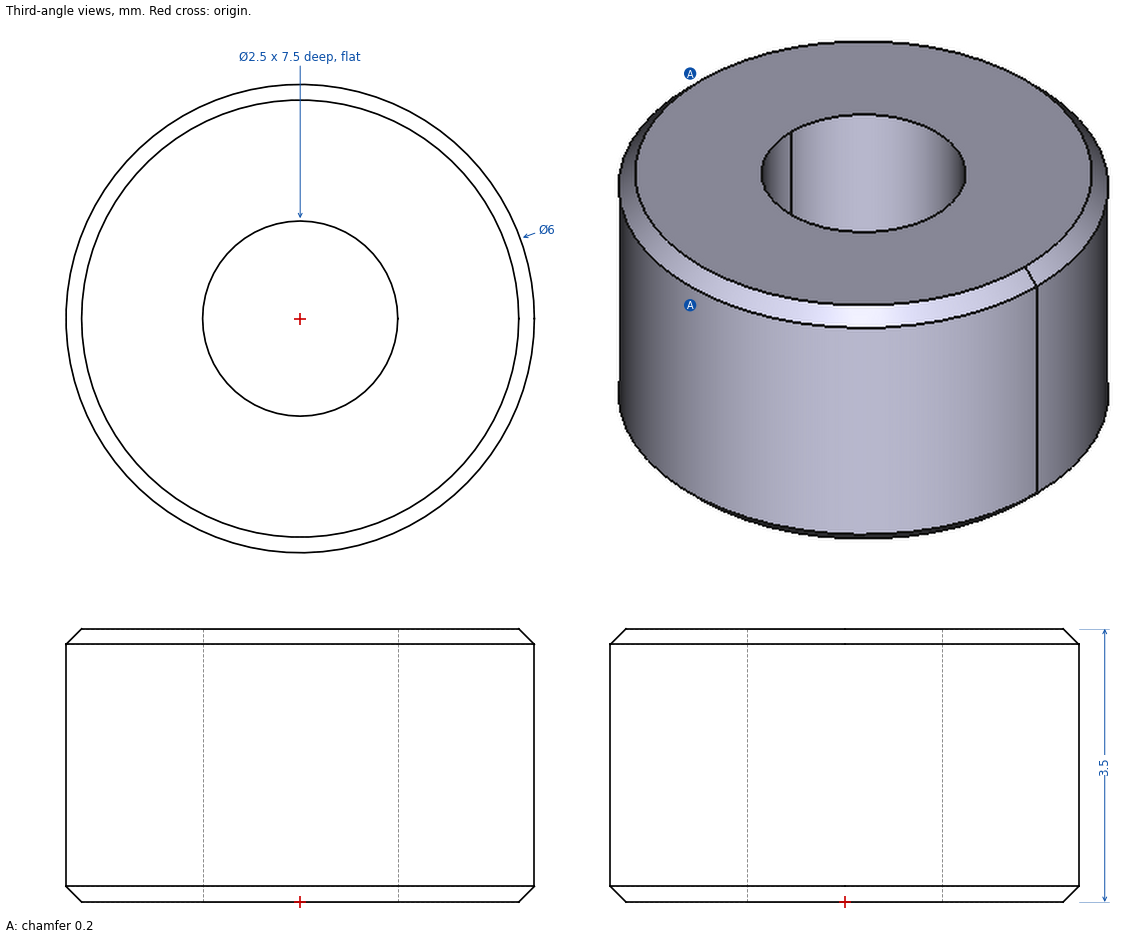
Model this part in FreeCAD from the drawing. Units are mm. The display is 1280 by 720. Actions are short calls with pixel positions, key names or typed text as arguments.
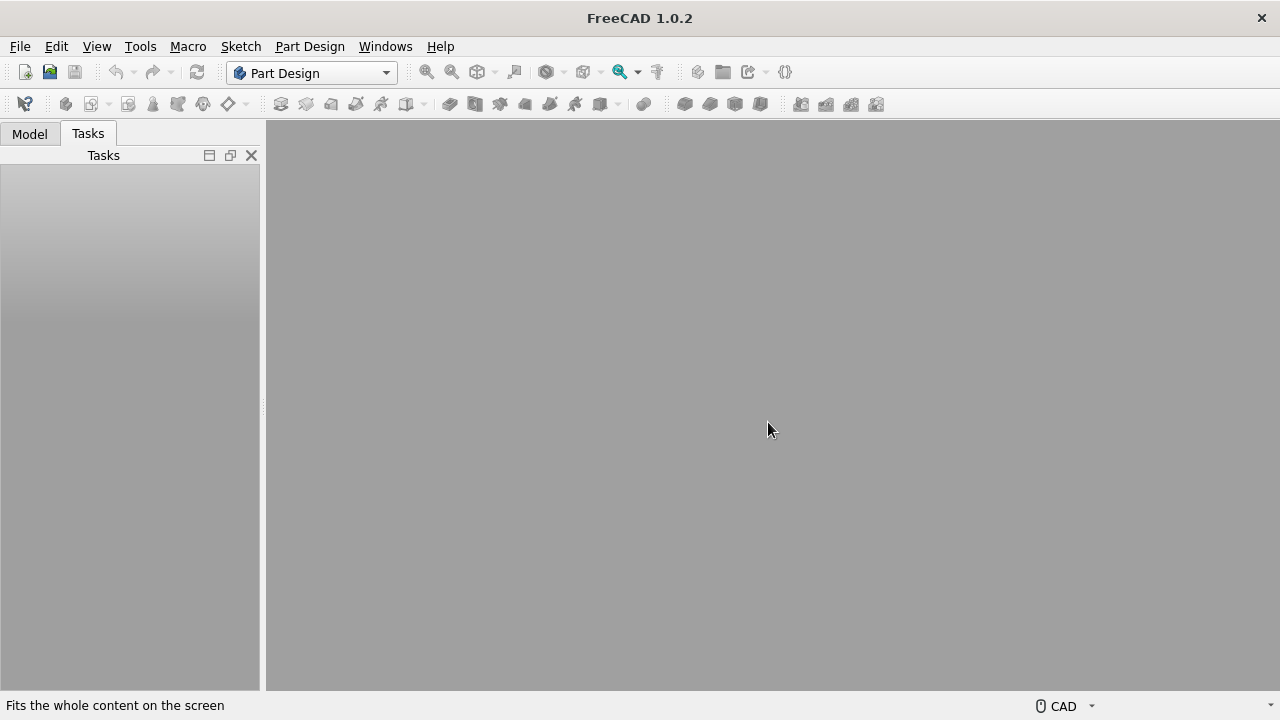
key(ctrl+n)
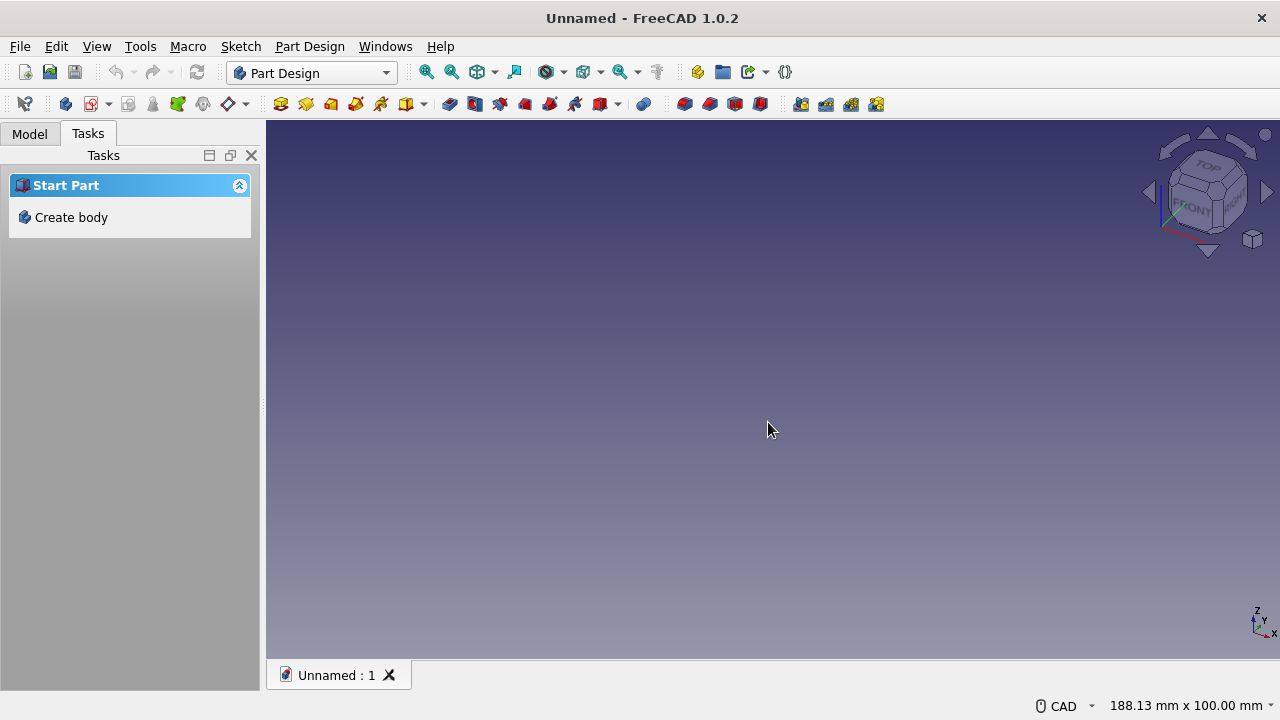
click(90, 104)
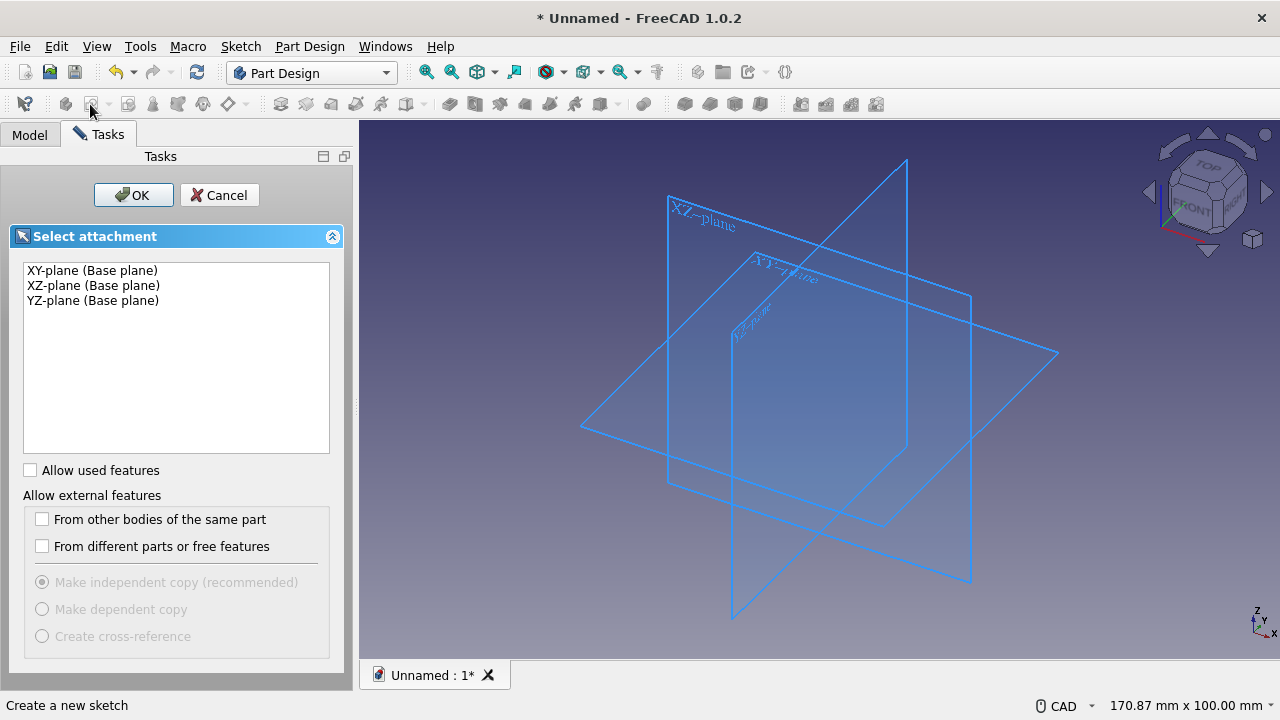
click(84, 270)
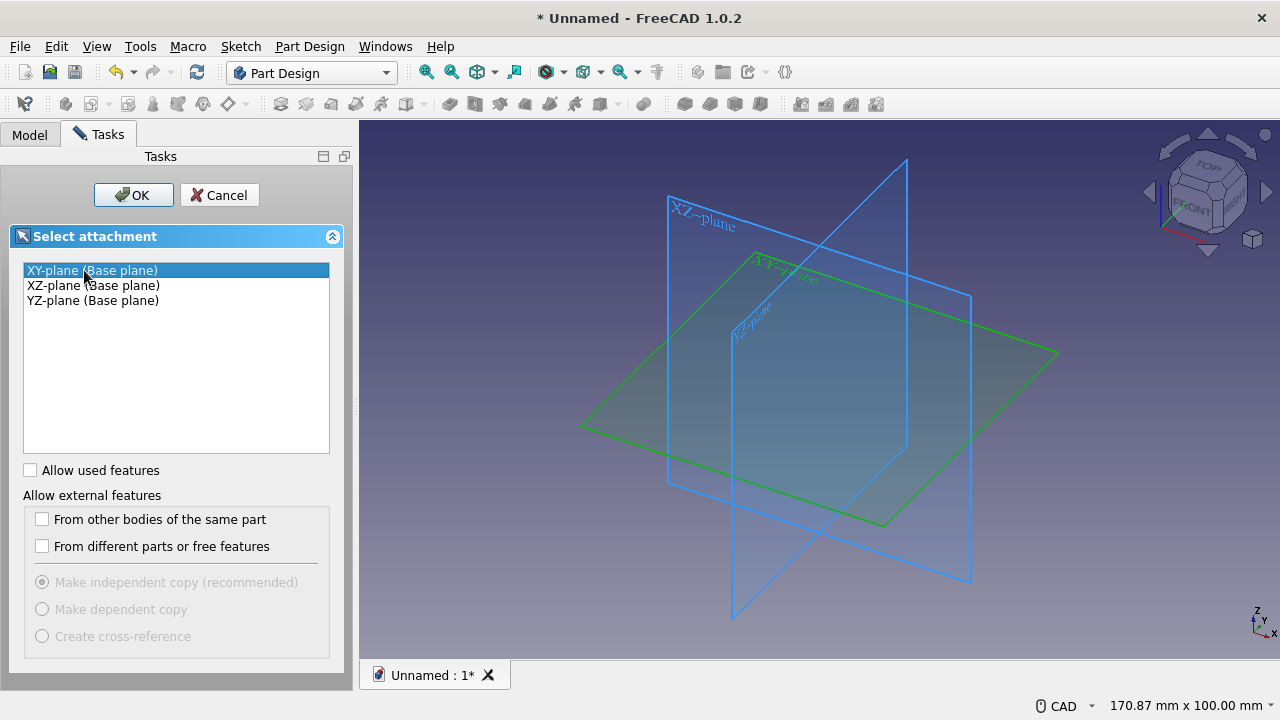
click(134, 195)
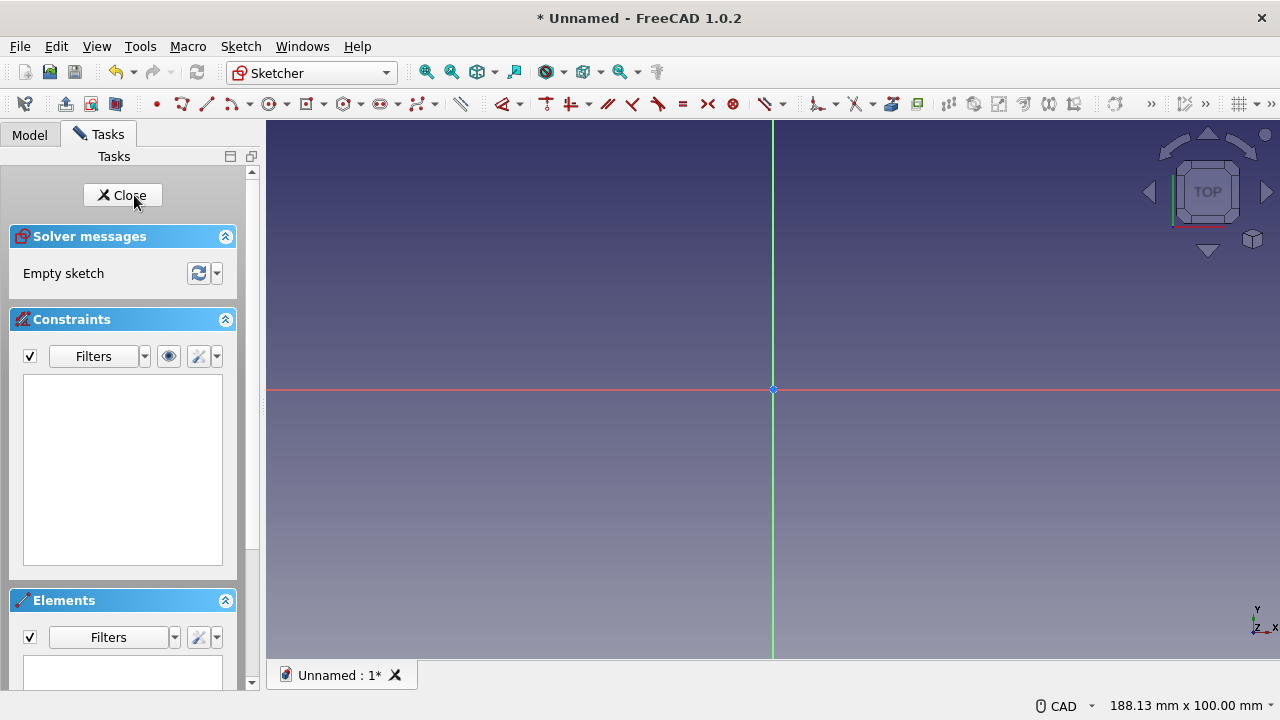
scroll(780, 390, up, 12)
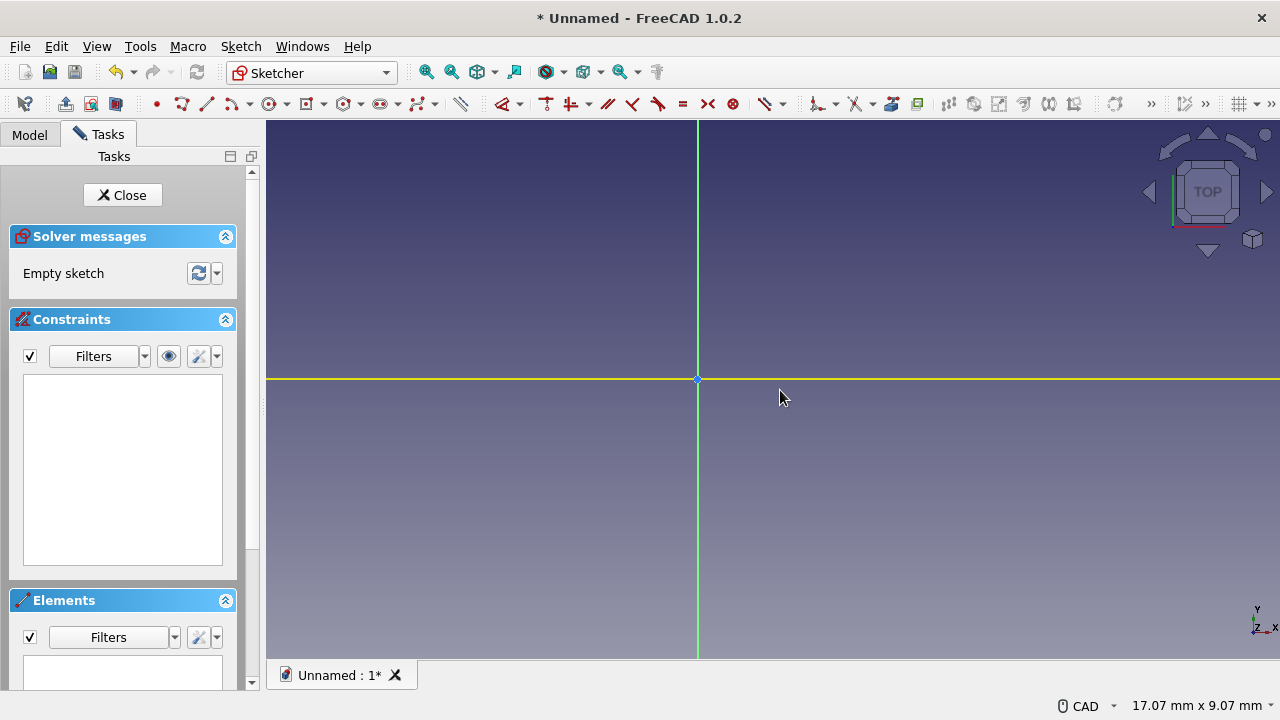
click(268, 104)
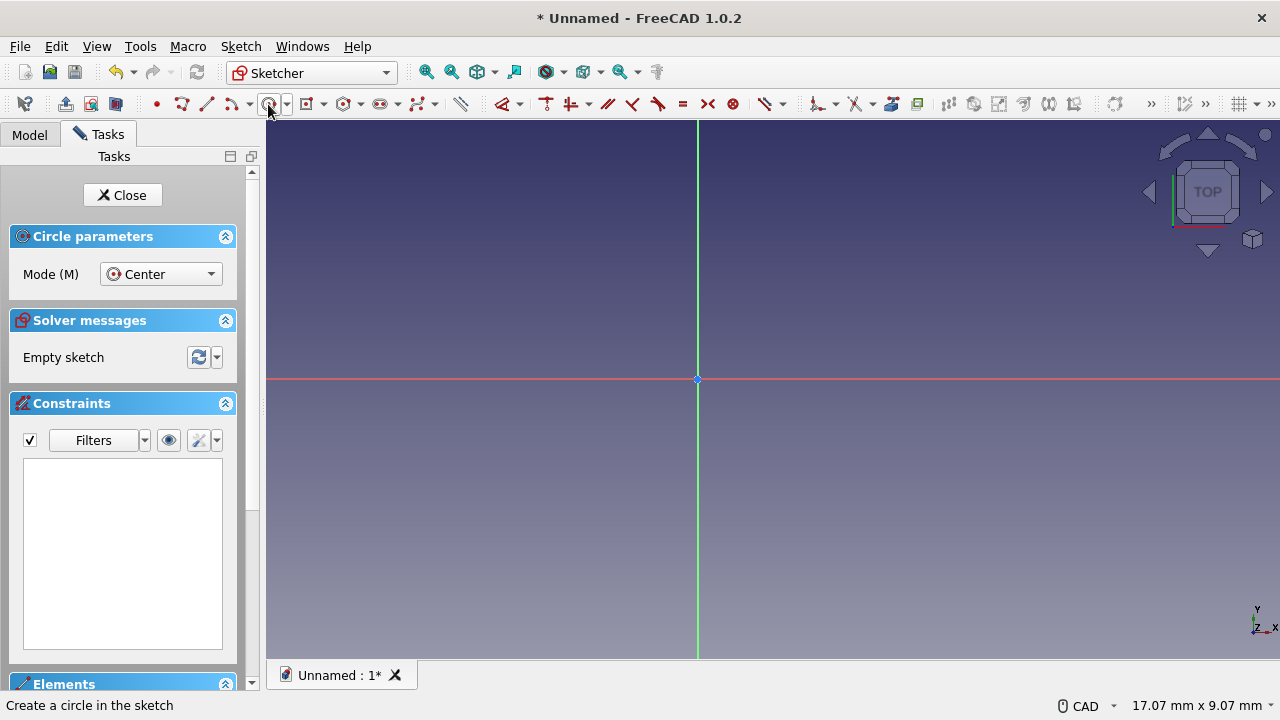
click(698, 379)
click(824, 253)
key(Escape)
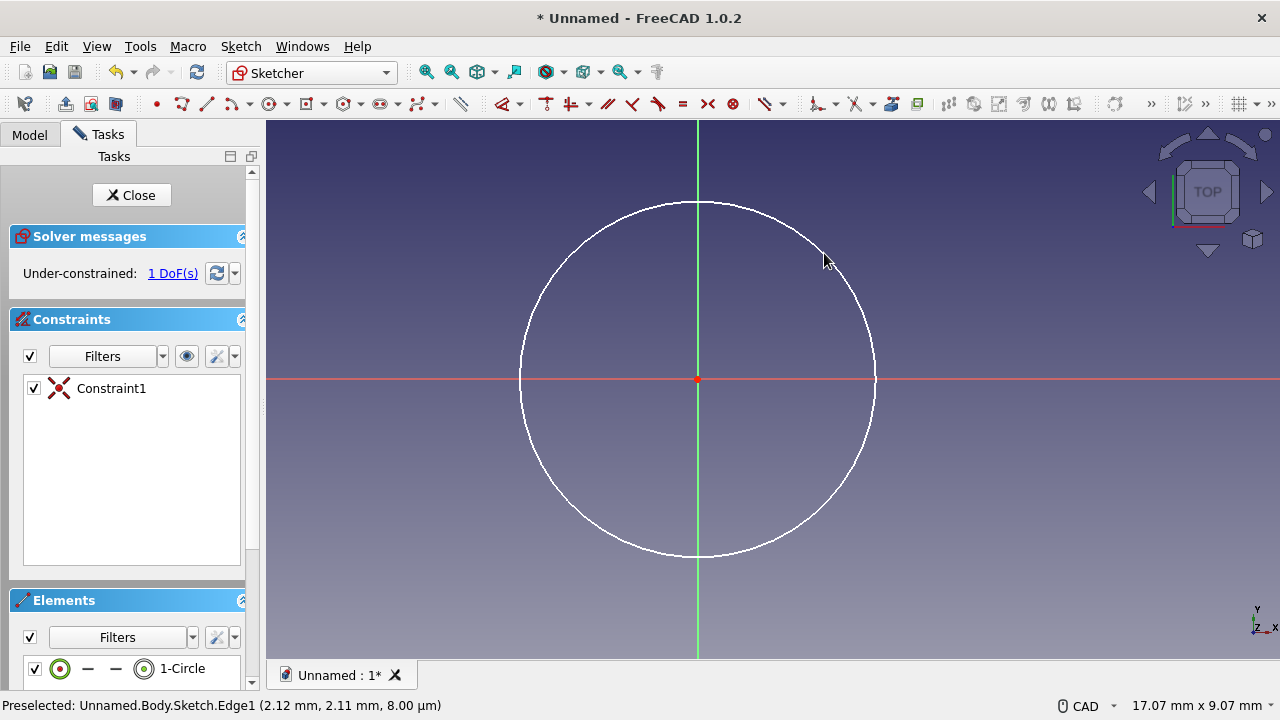
key(d)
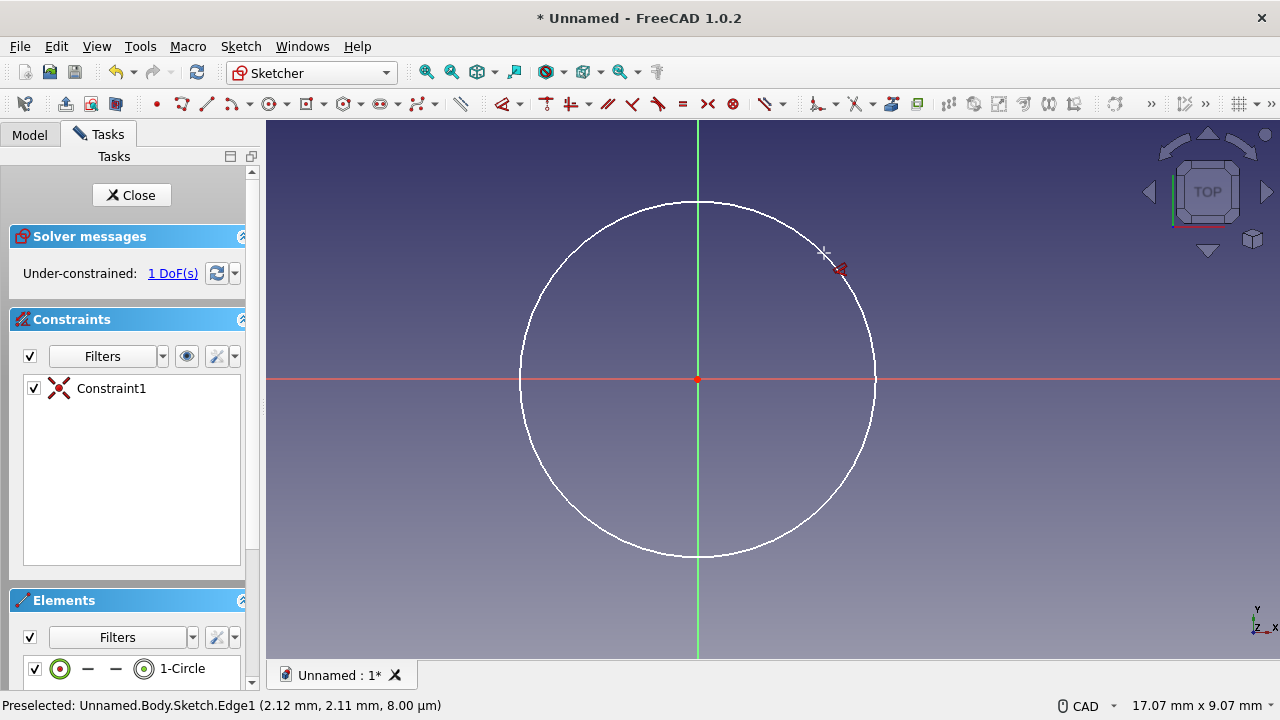
click(823, 253)
click(846, 230)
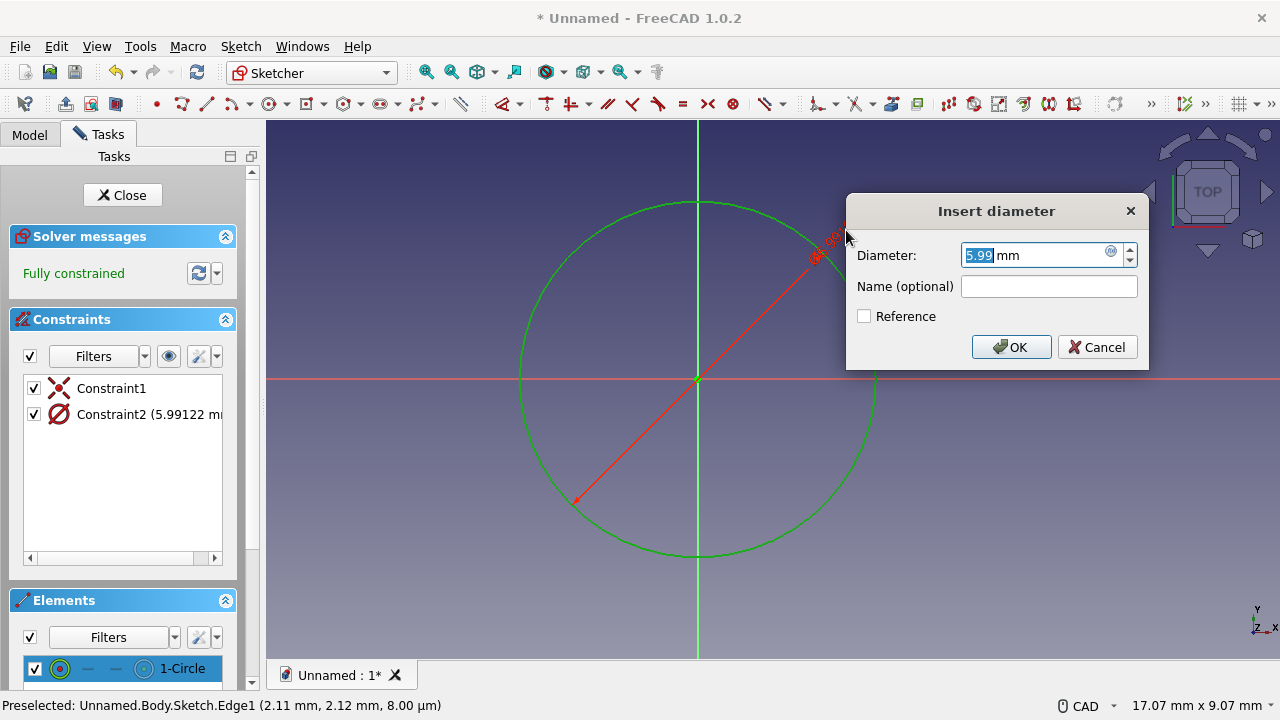
text(6)
key(Return)
key(Escape)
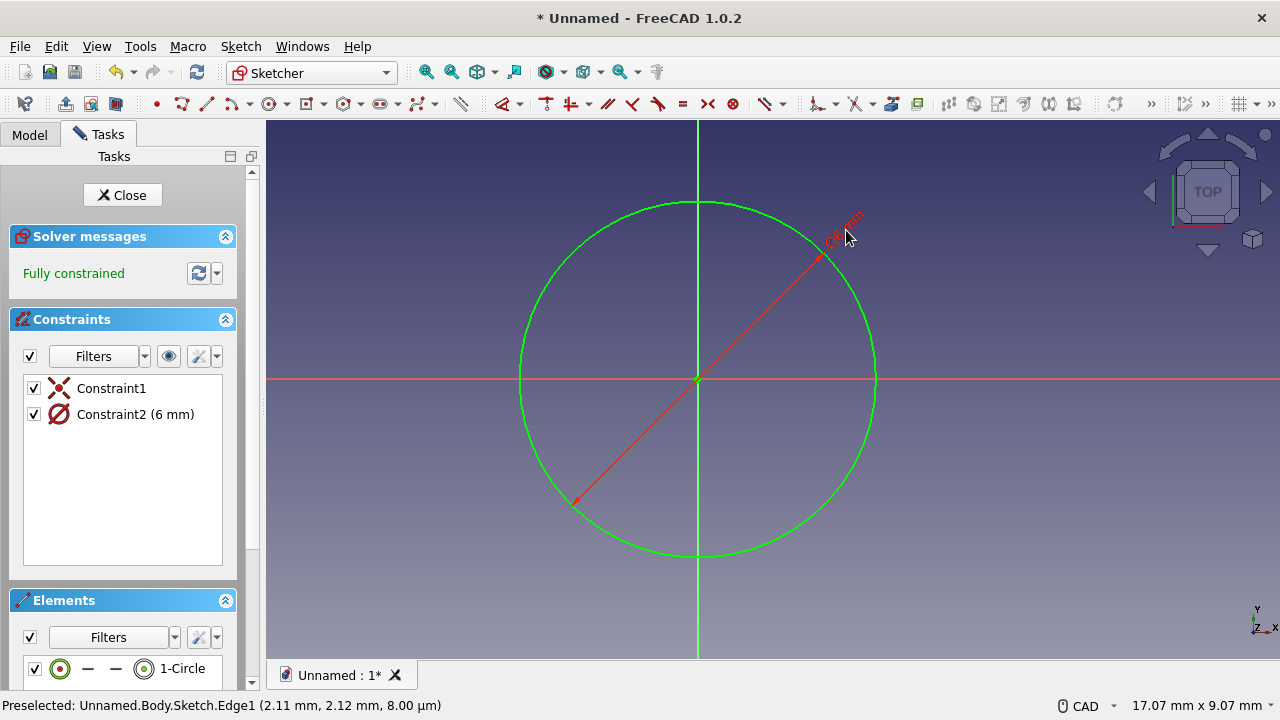
click(123, 195)